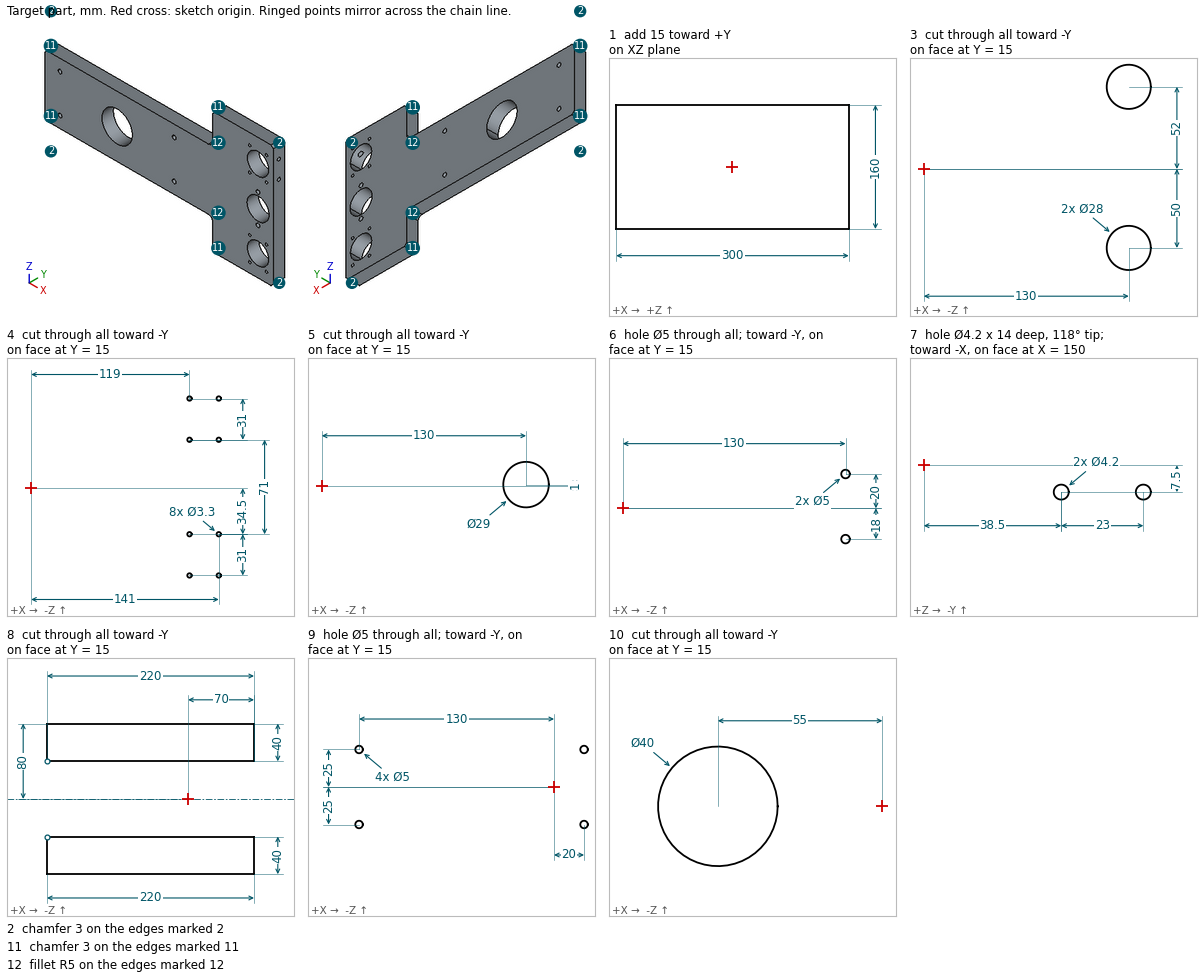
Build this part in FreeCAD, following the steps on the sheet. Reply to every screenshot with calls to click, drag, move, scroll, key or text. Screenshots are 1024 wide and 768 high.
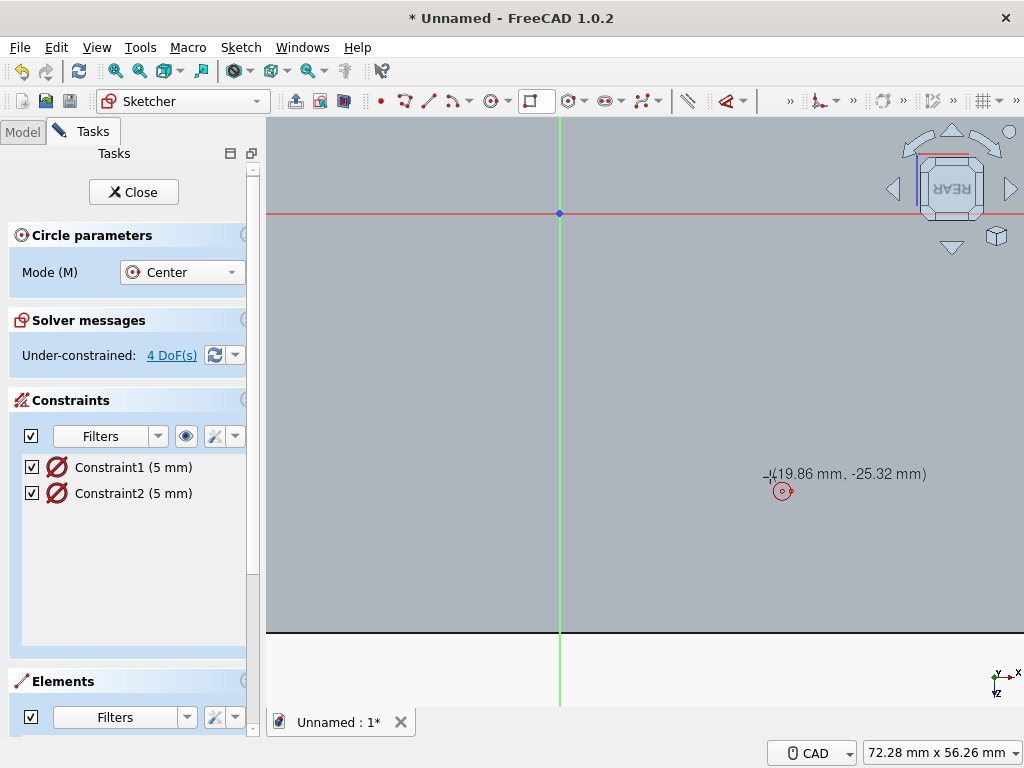
scroll(771, 477, down, 7)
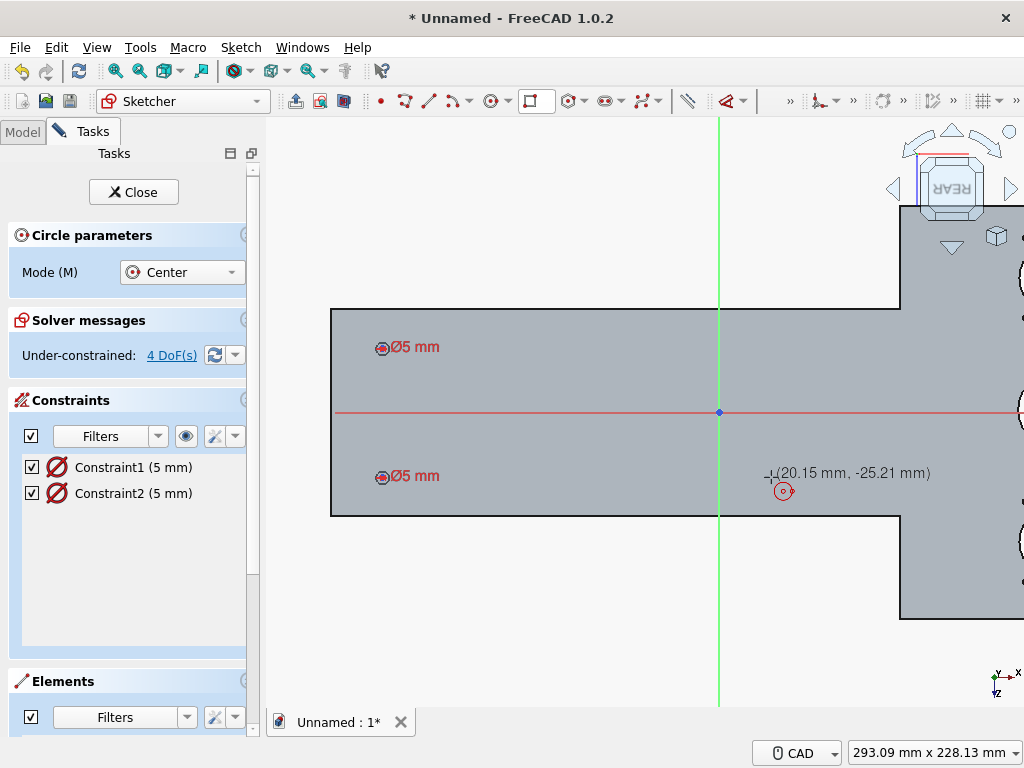
click(771, 477)
move(776, 473)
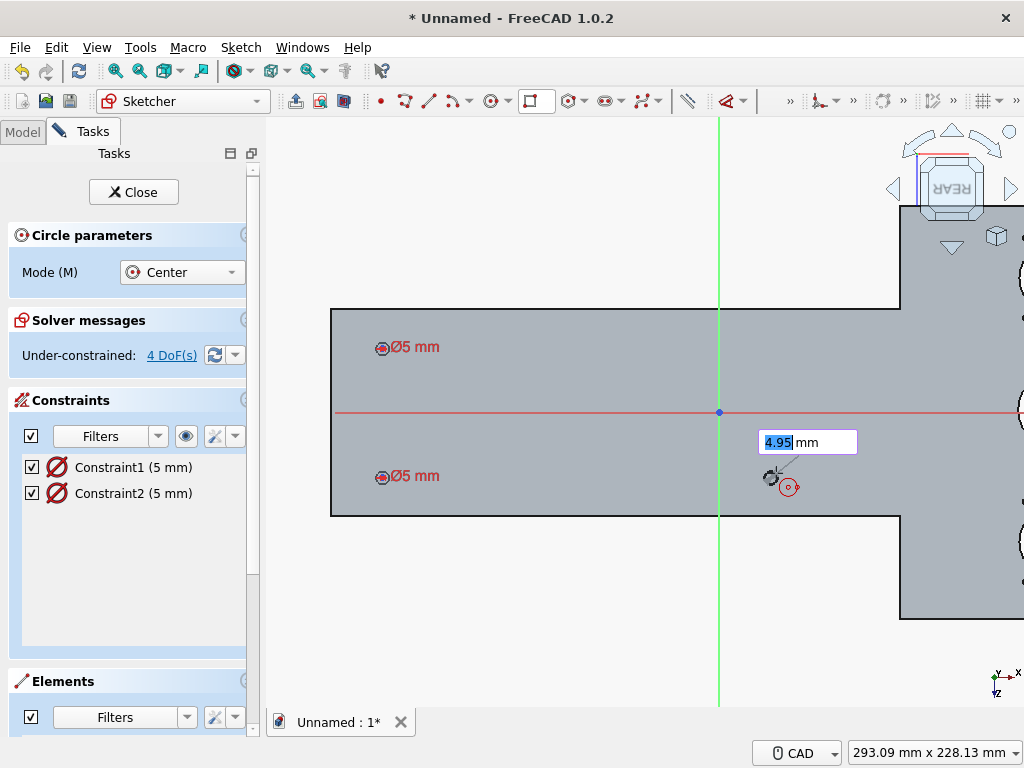
text(5)
key(Return)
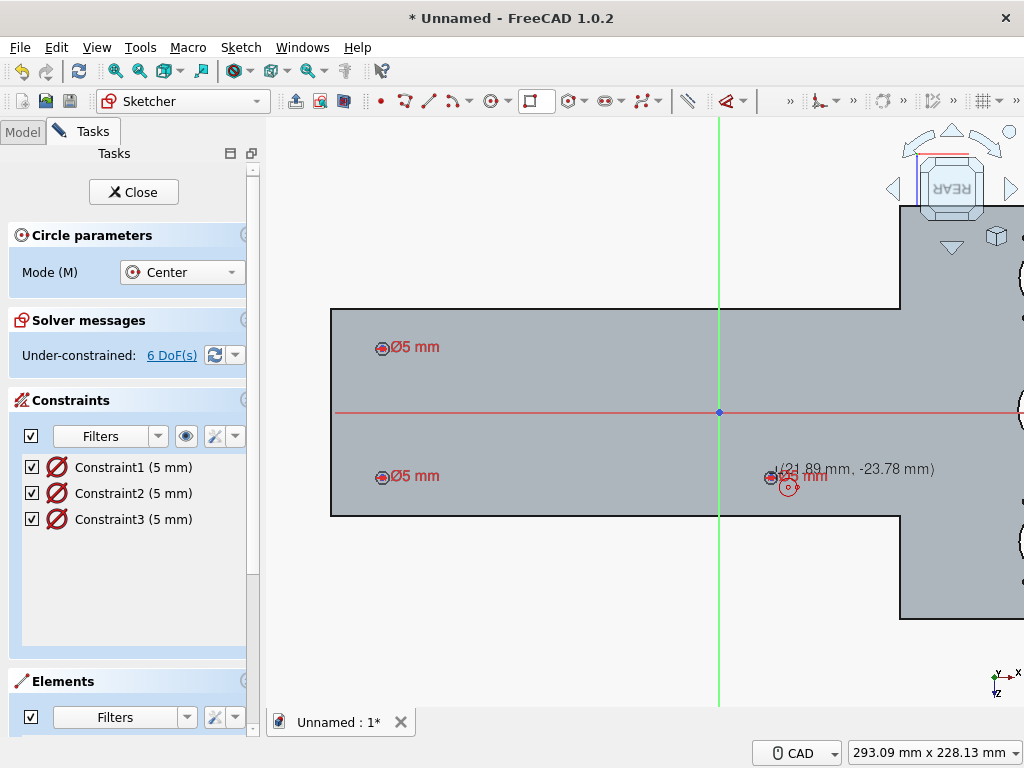
scroll(771, 348, up, 7)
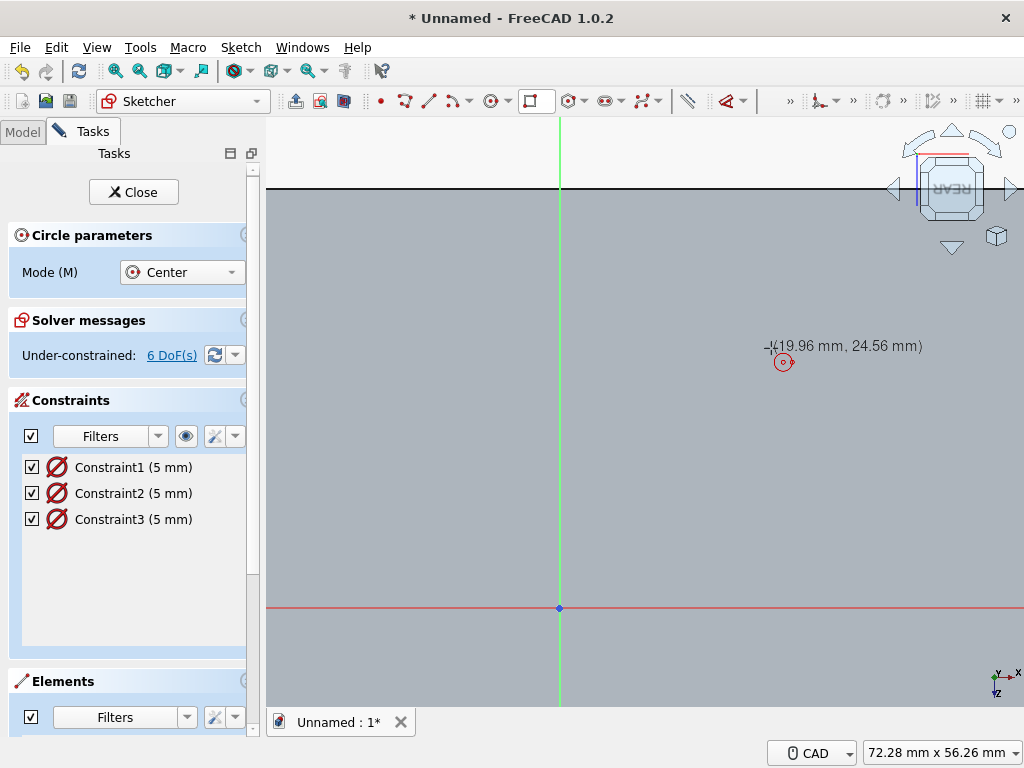
scroll(771, 348, down, 7)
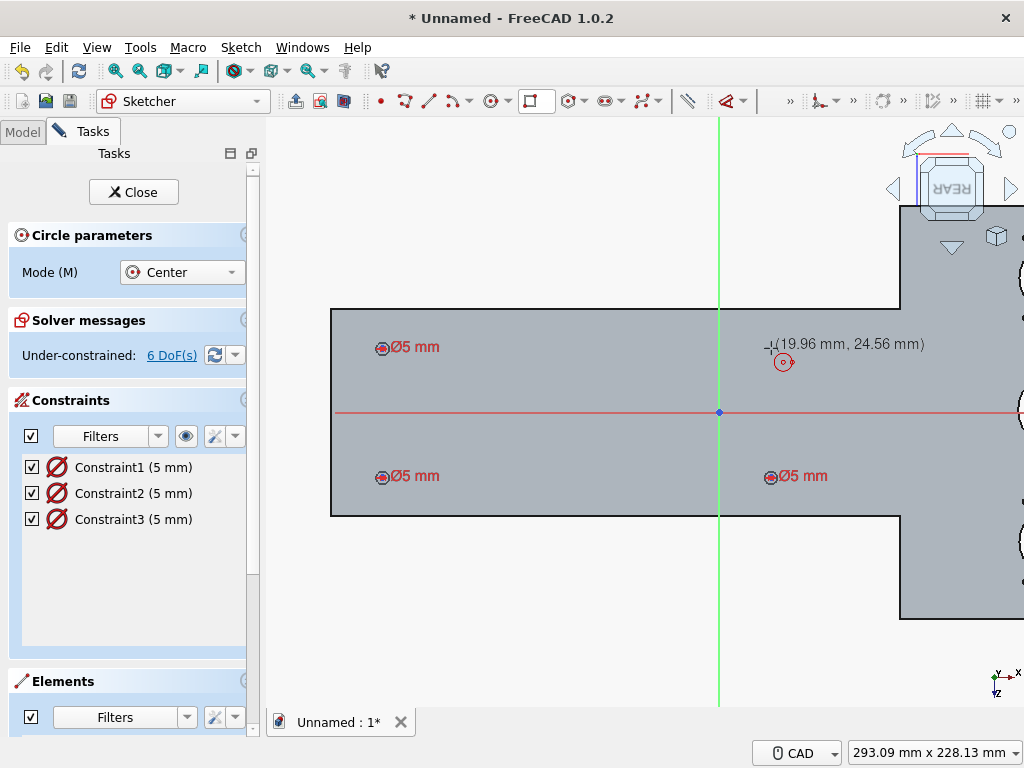
click(771, 348)
move(776, 343)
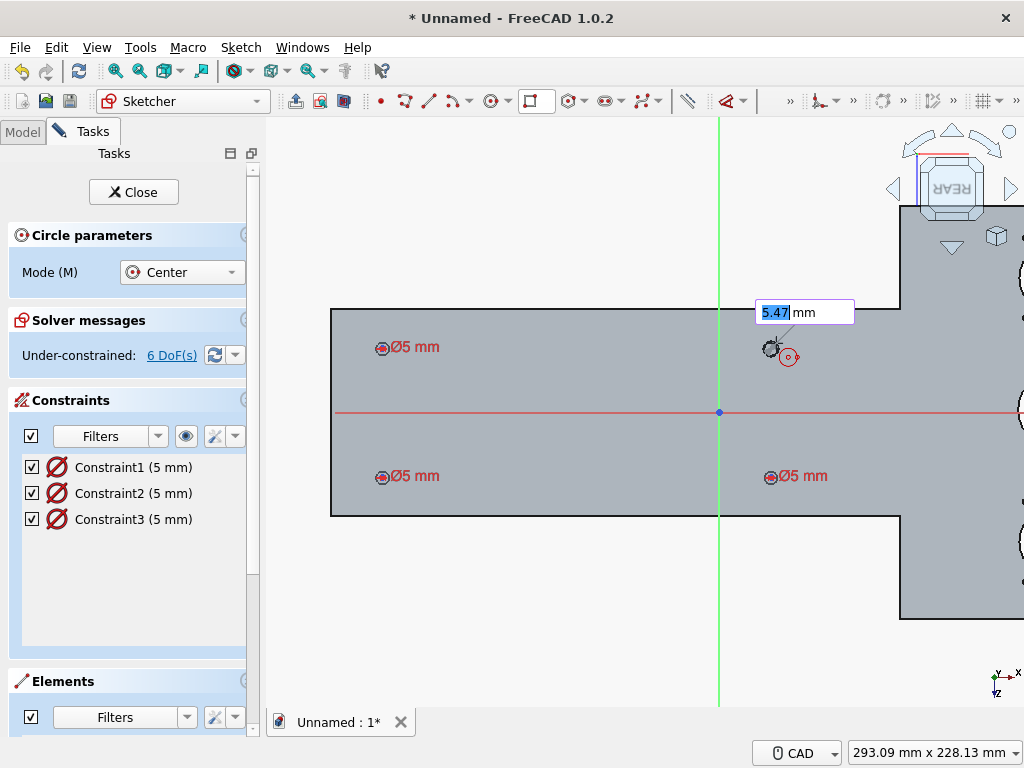
text(5)
key(Return)
key(Escape)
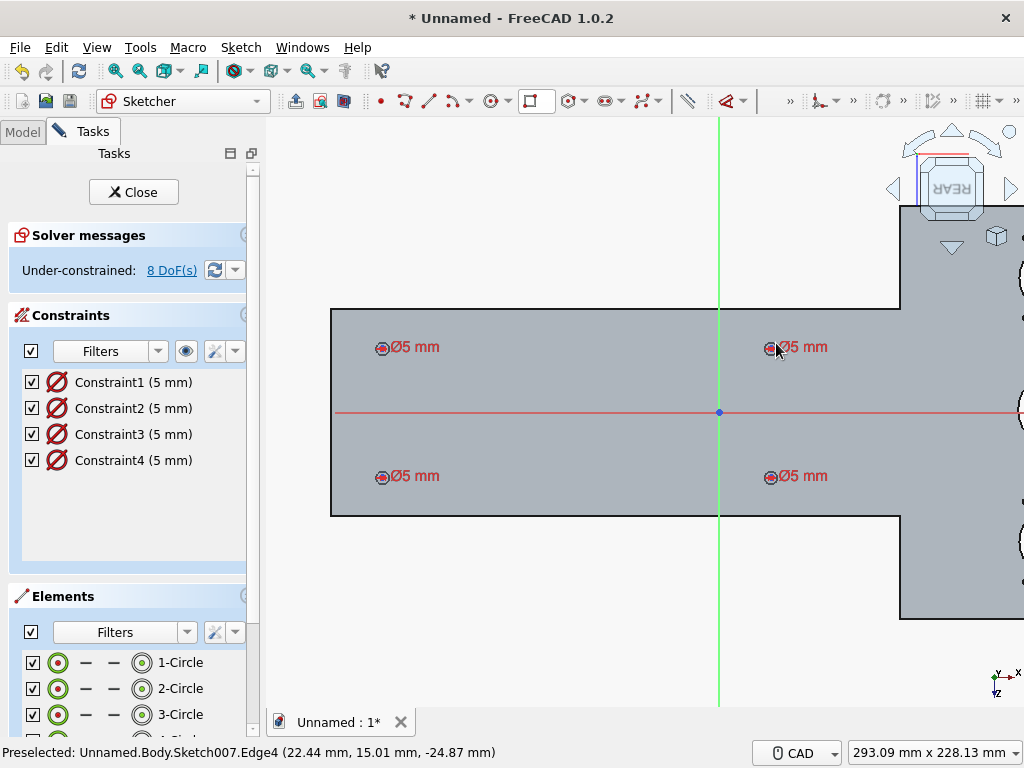
click(383, 349)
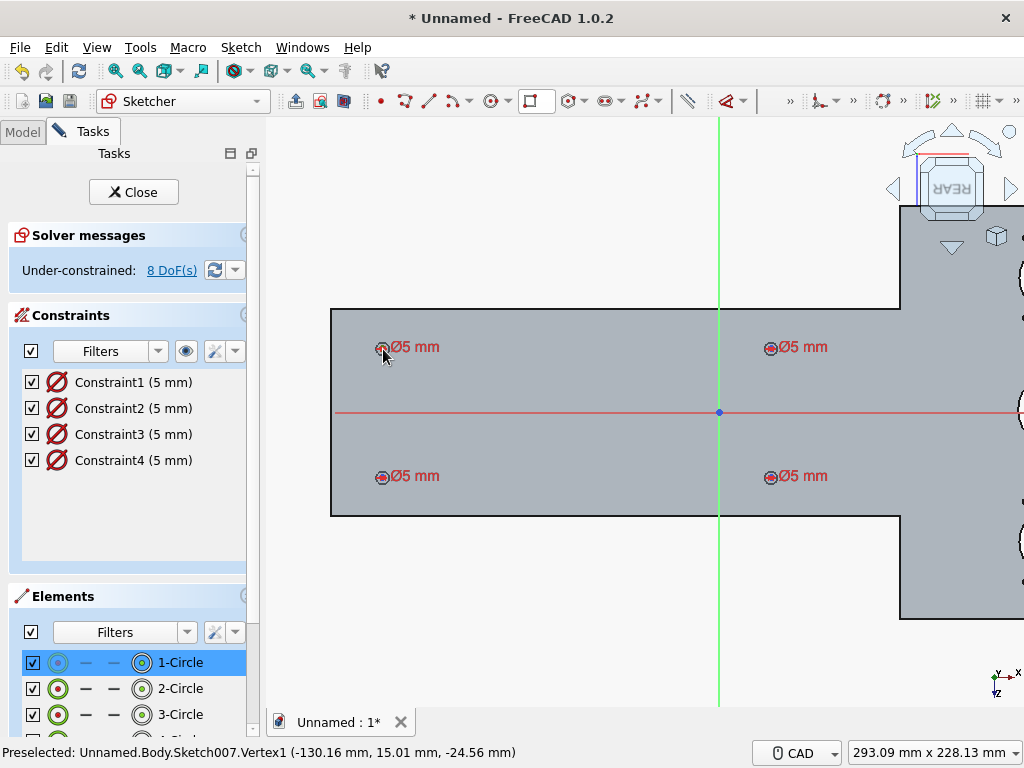
click(383, 478)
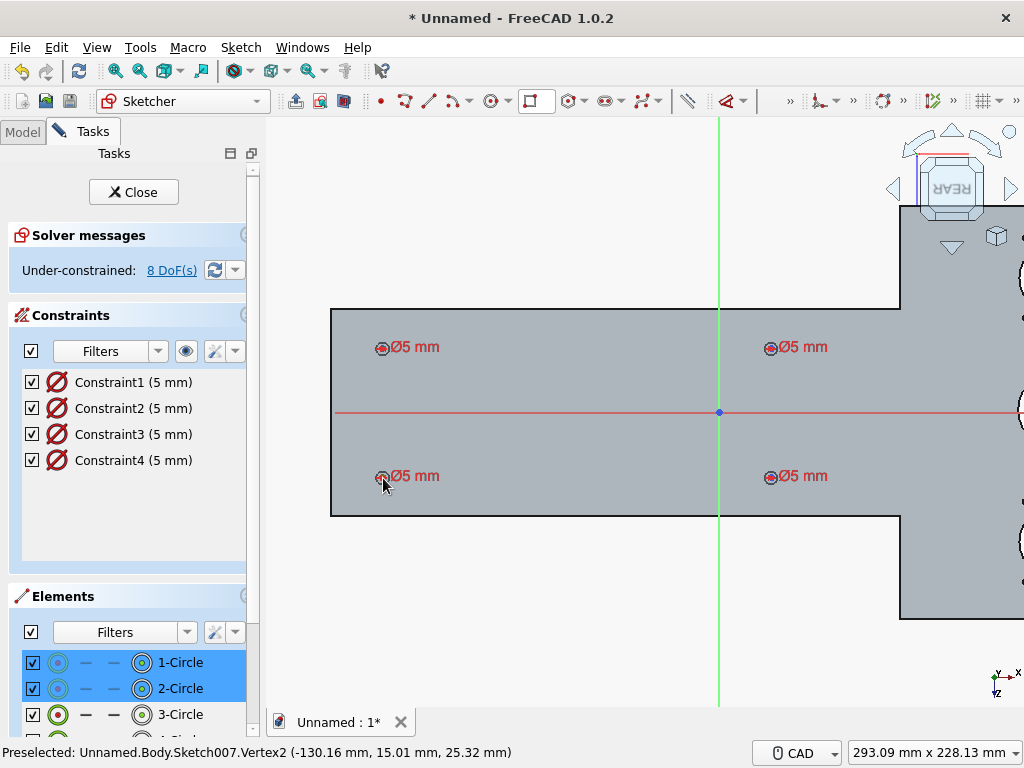
key(v)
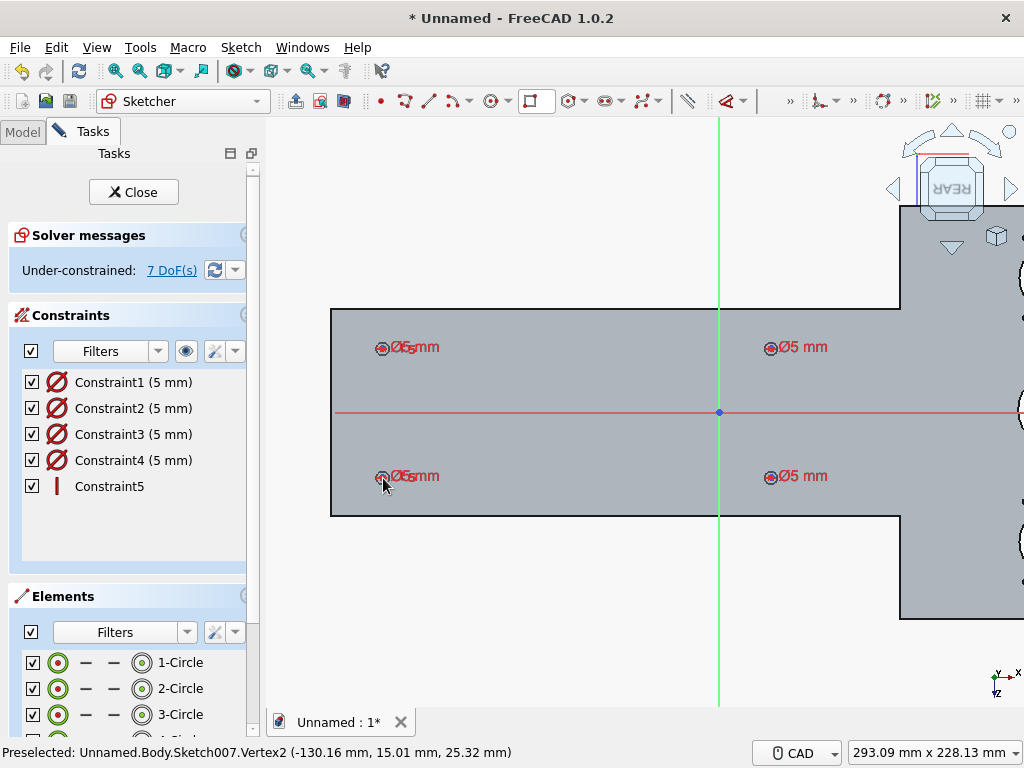
click(383, 478)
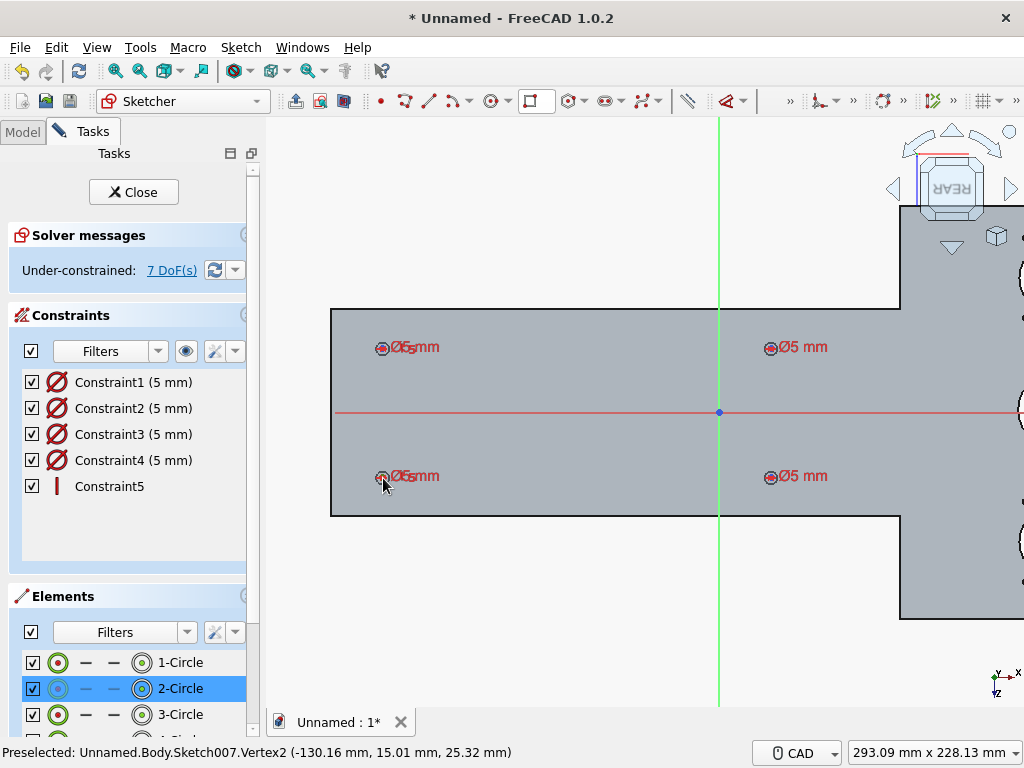
click(771, 478)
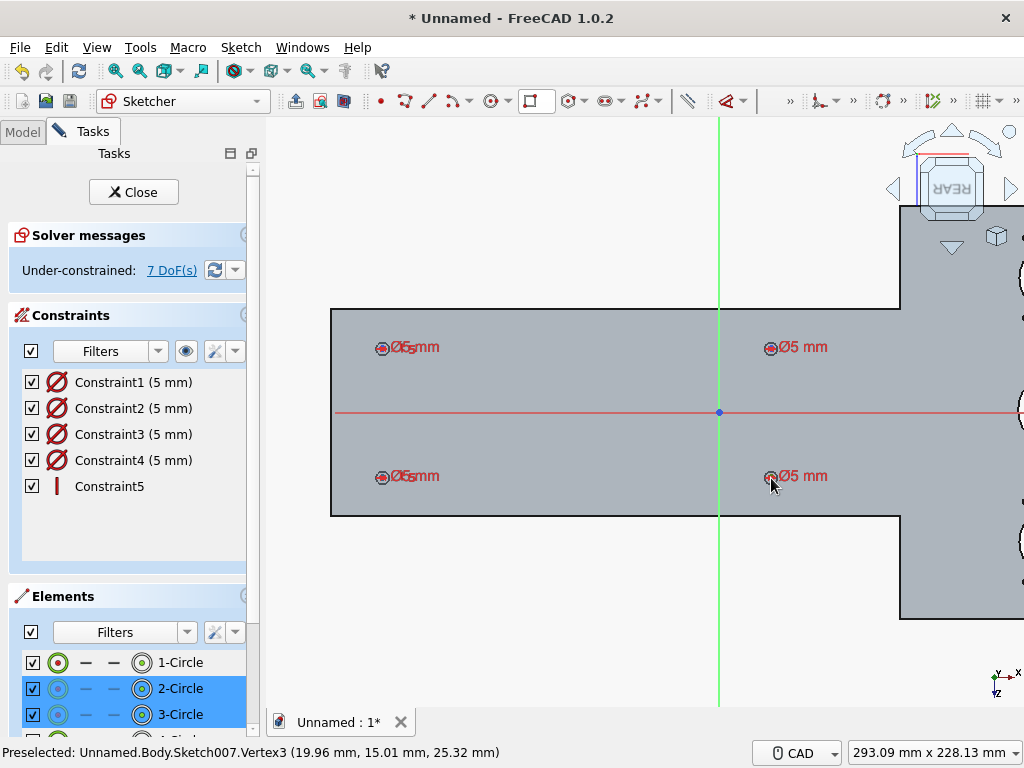
key(h)